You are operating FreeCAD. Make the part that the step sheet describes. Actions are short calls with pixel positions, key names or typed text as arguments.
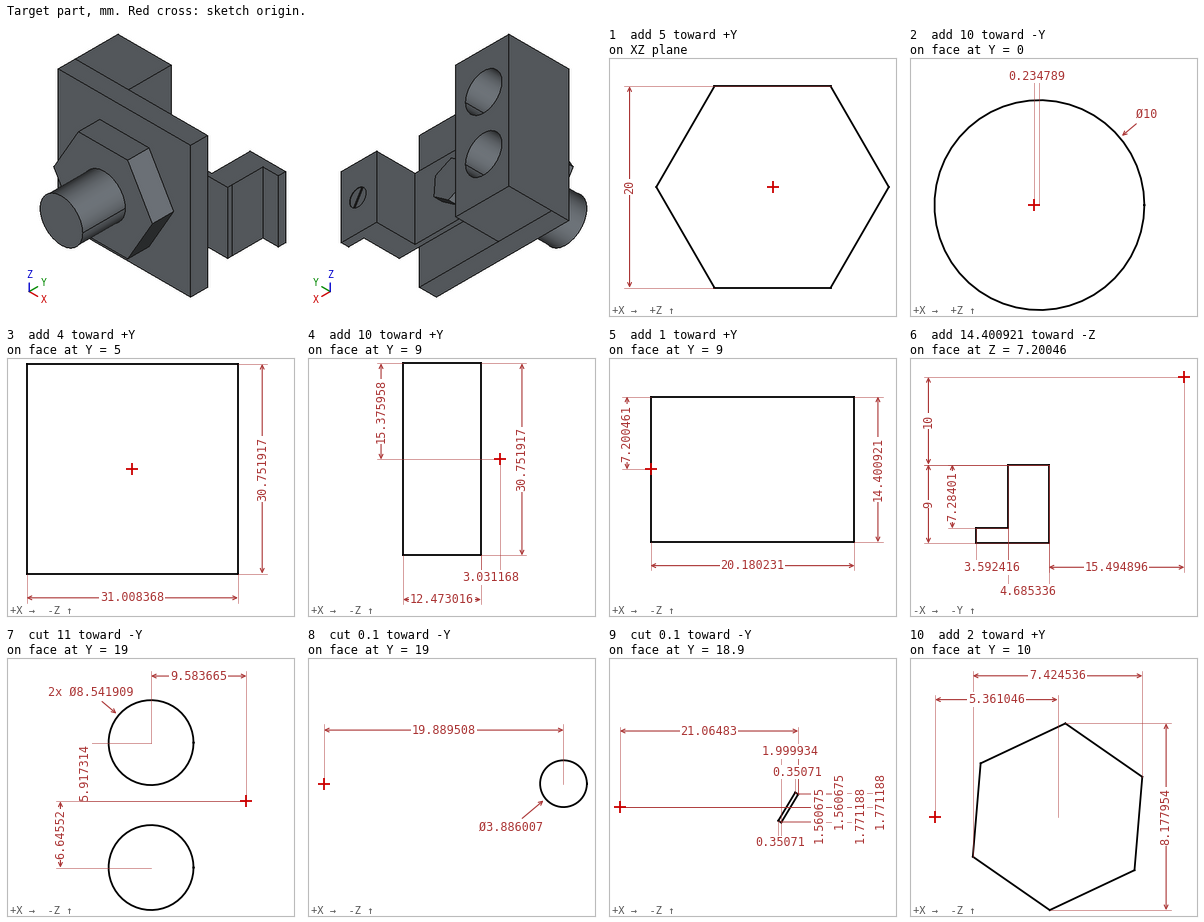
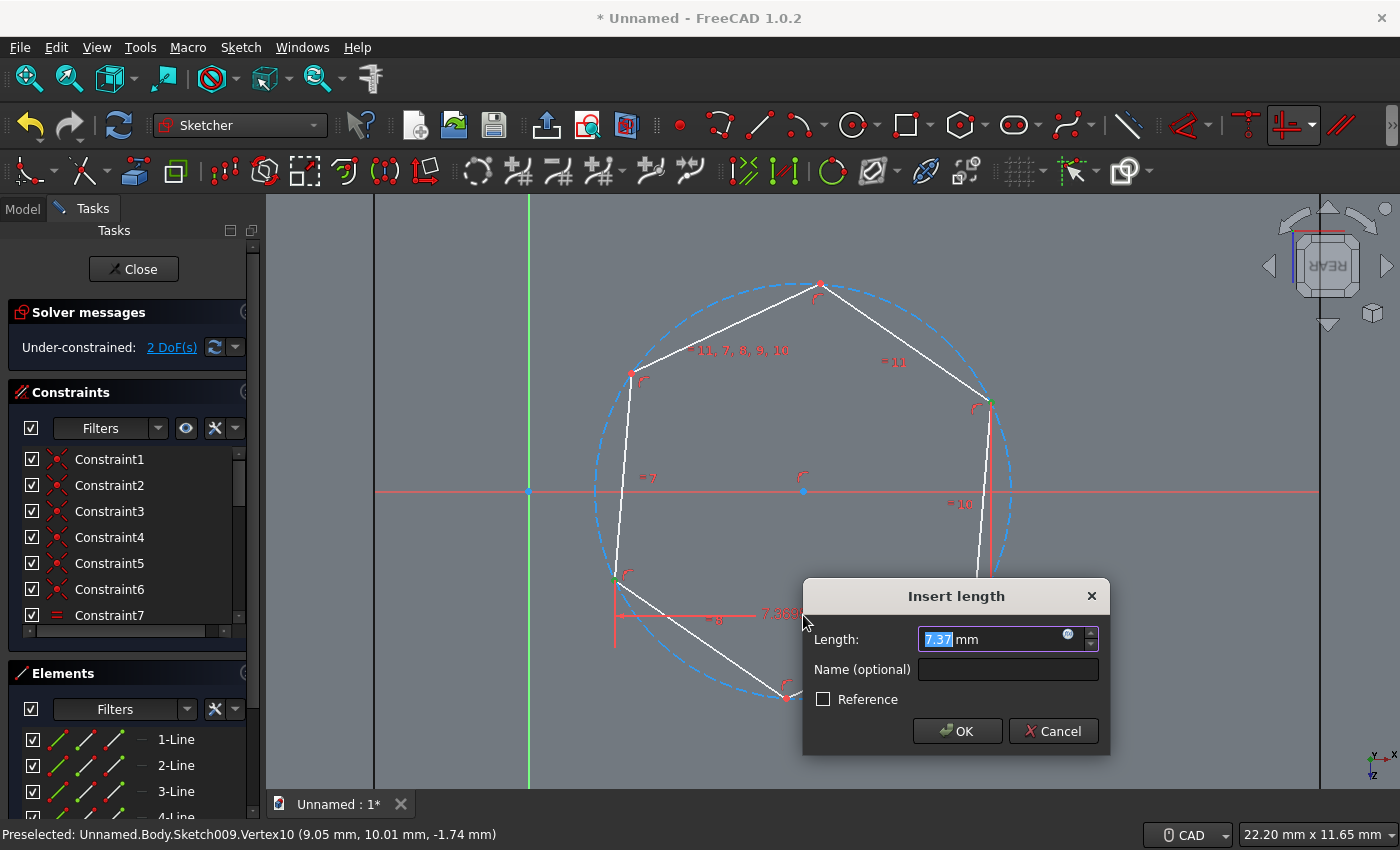
text(7.424536)
key(Return)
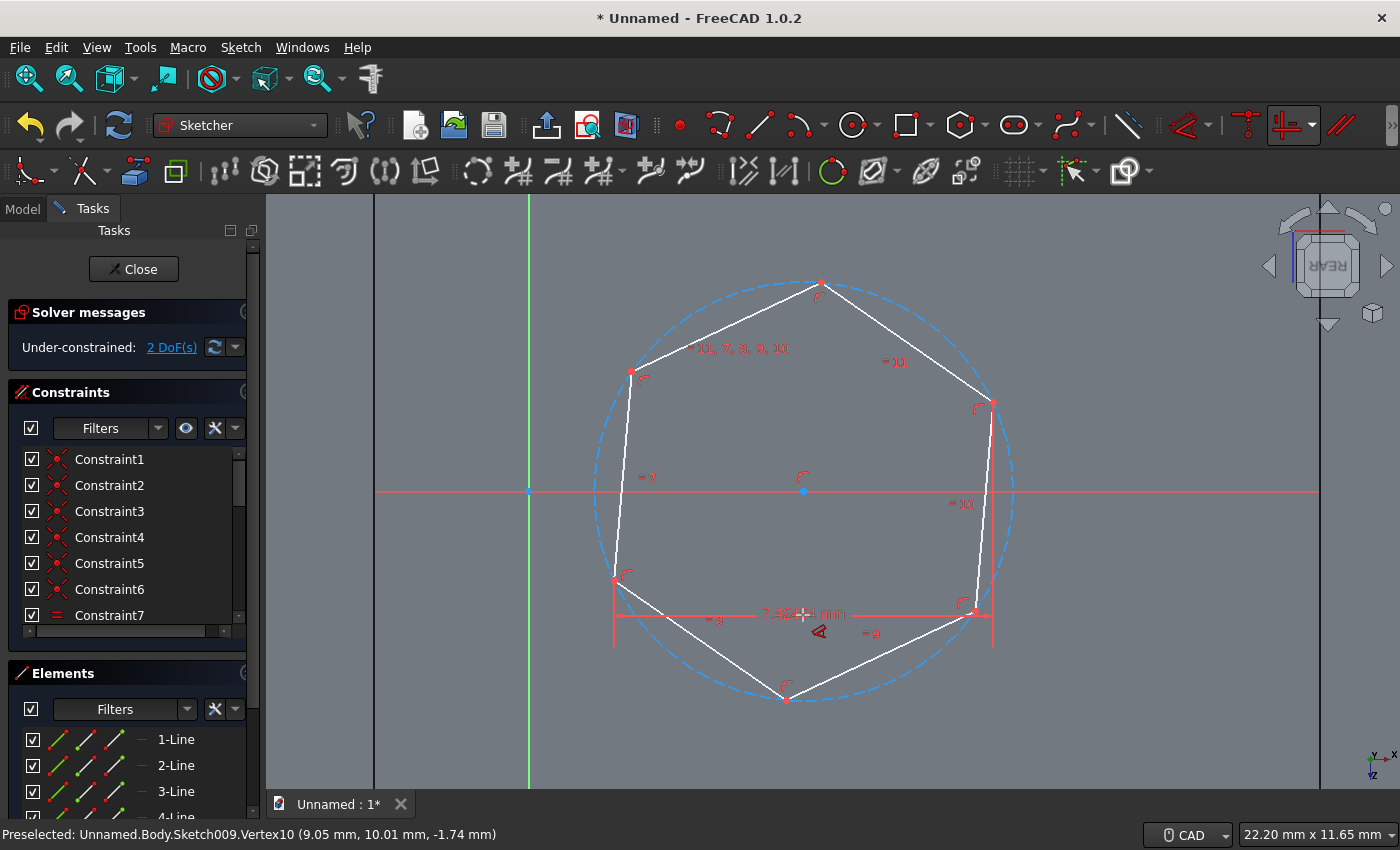
click(786, 700)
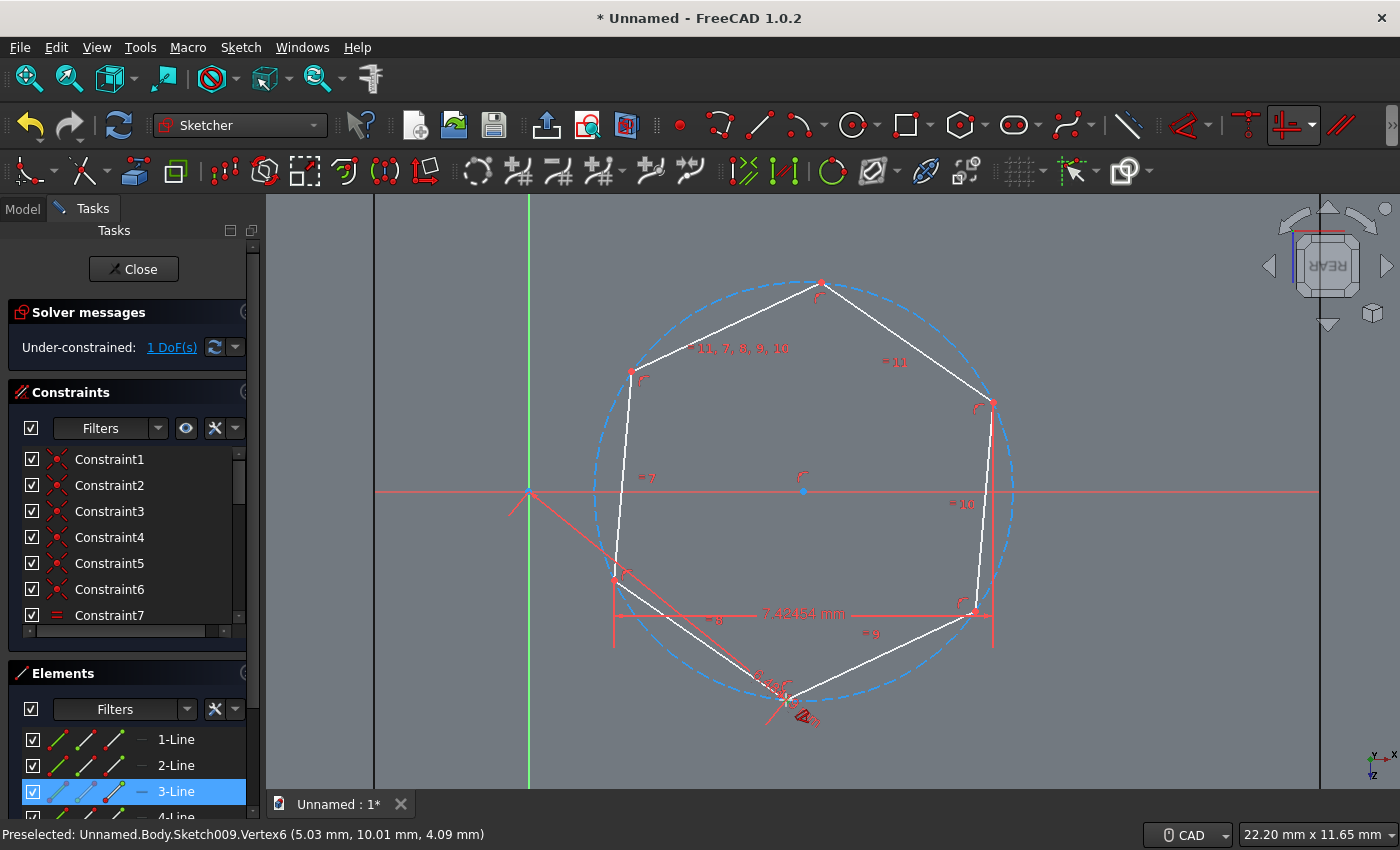
click(821, 283)
click(855, 395)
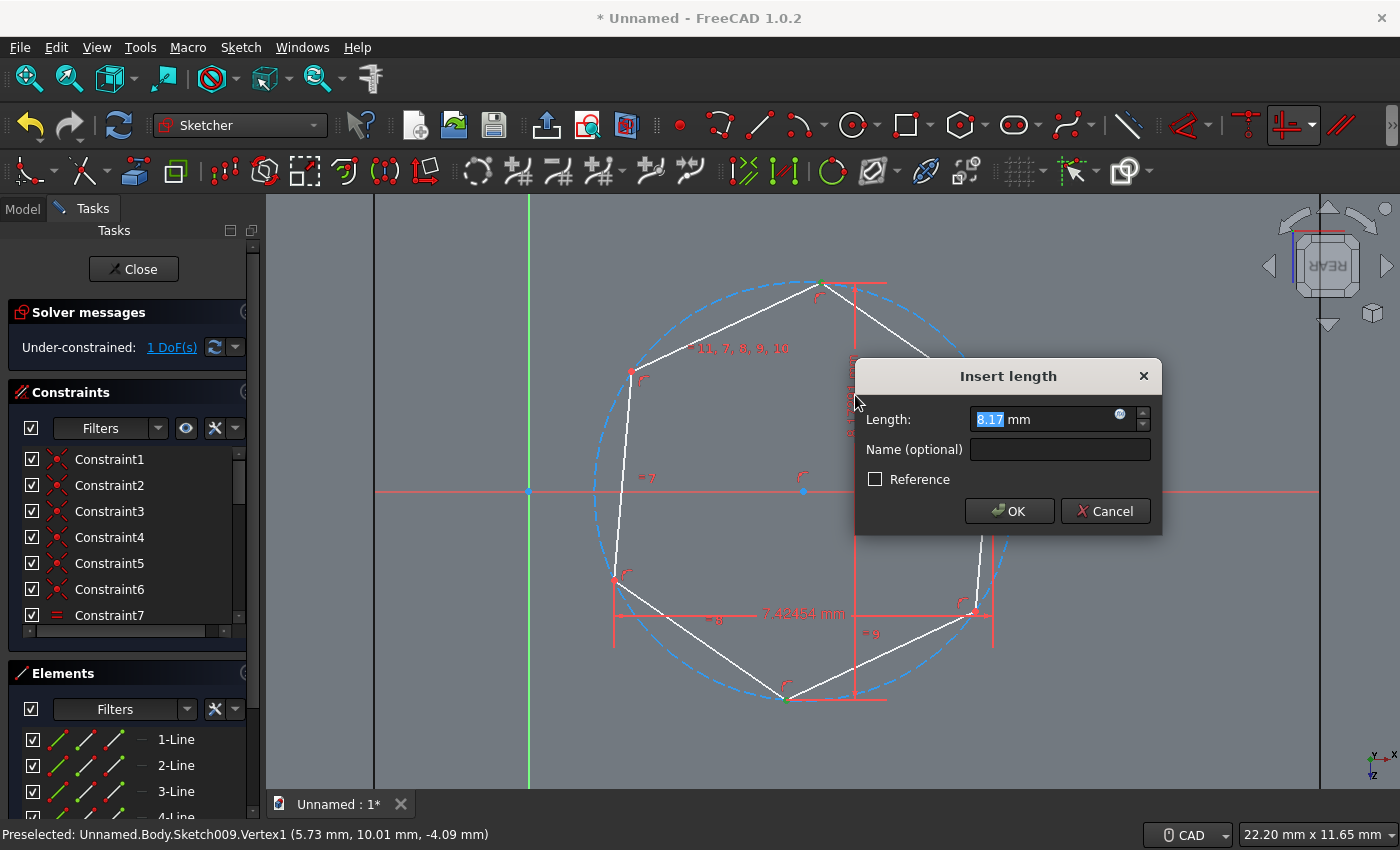
text(8.177954)
key(Return)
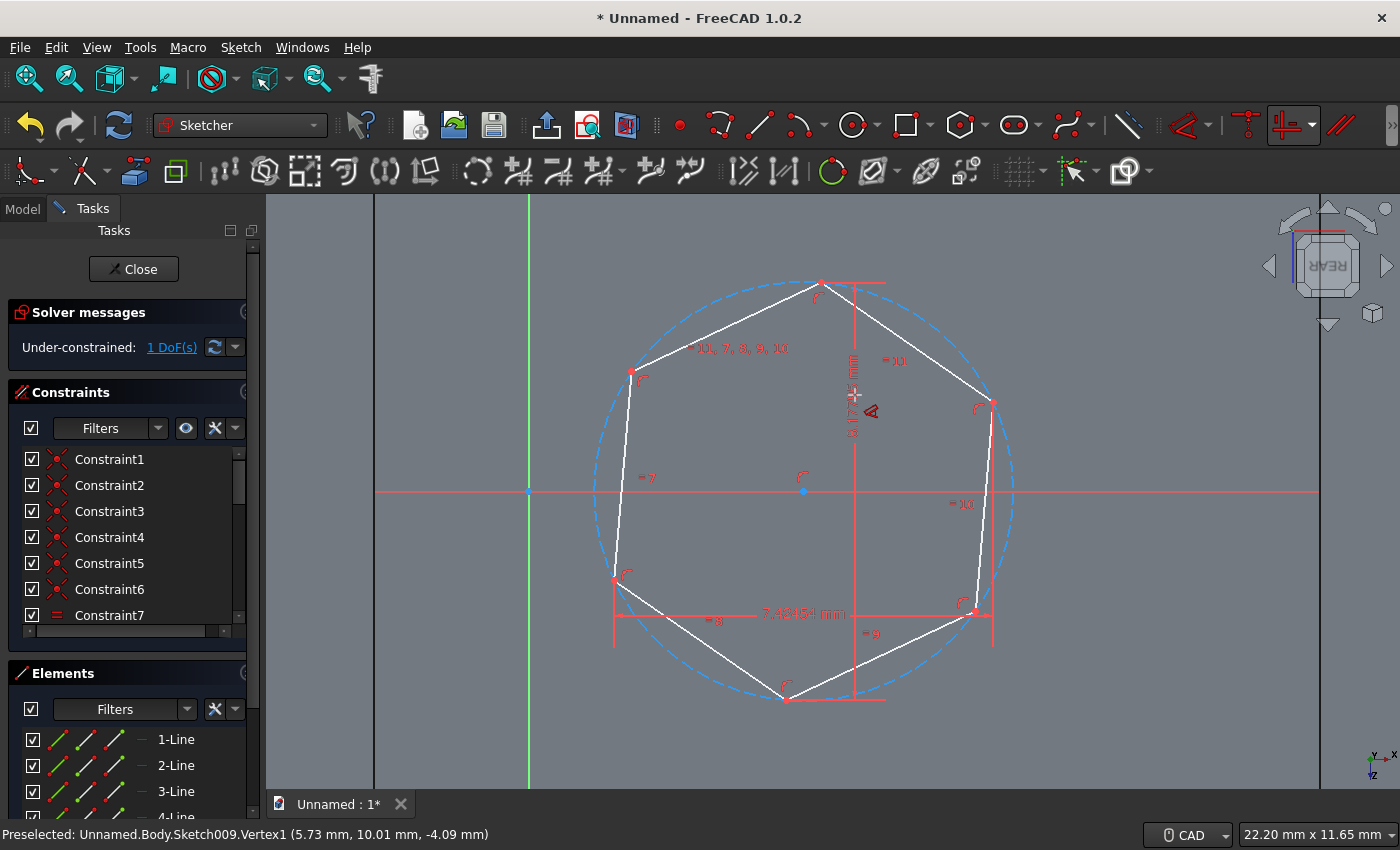
click(804, 491)
click(666, 525)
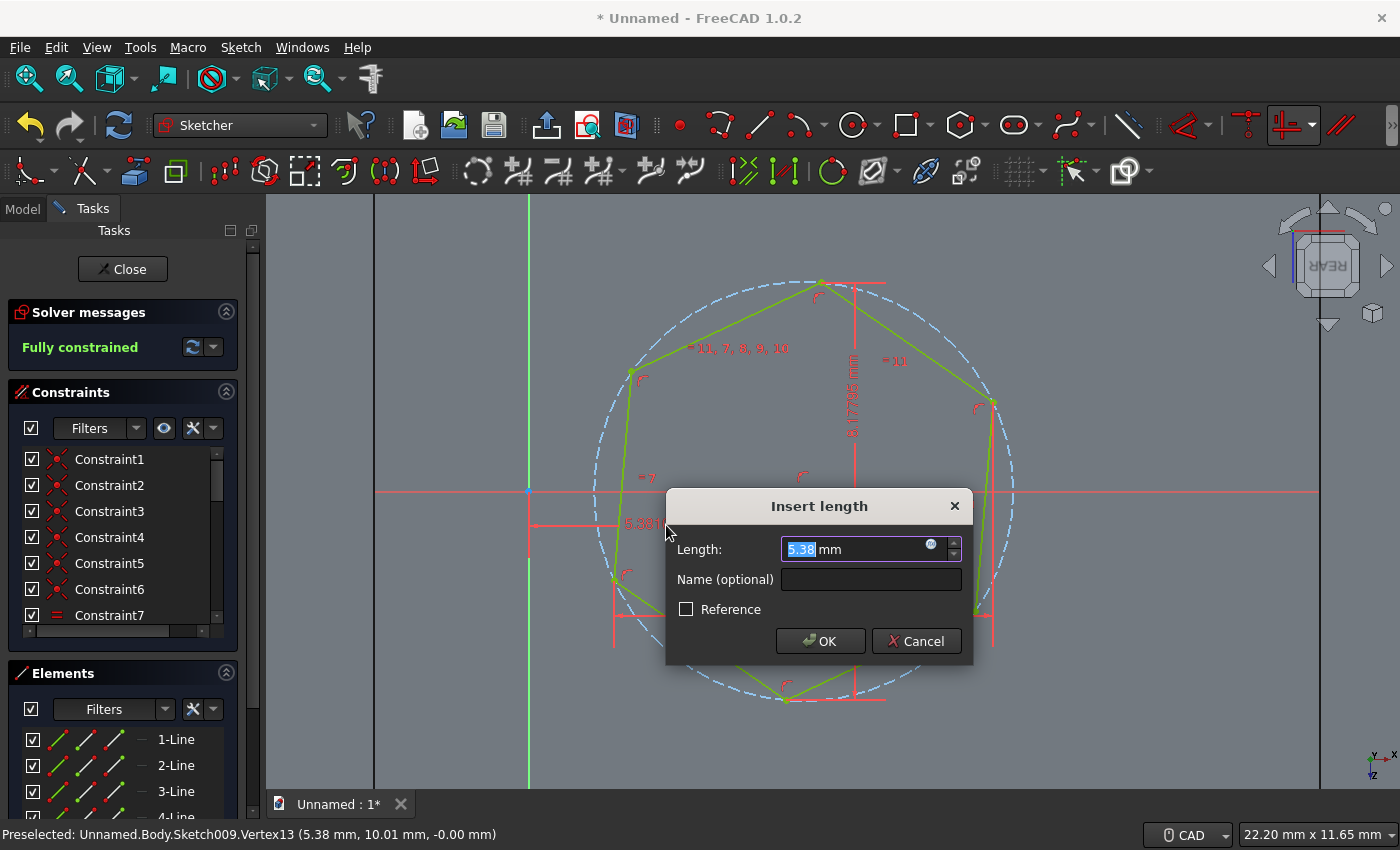
text(5.361046)
key(Return)
key(Escape)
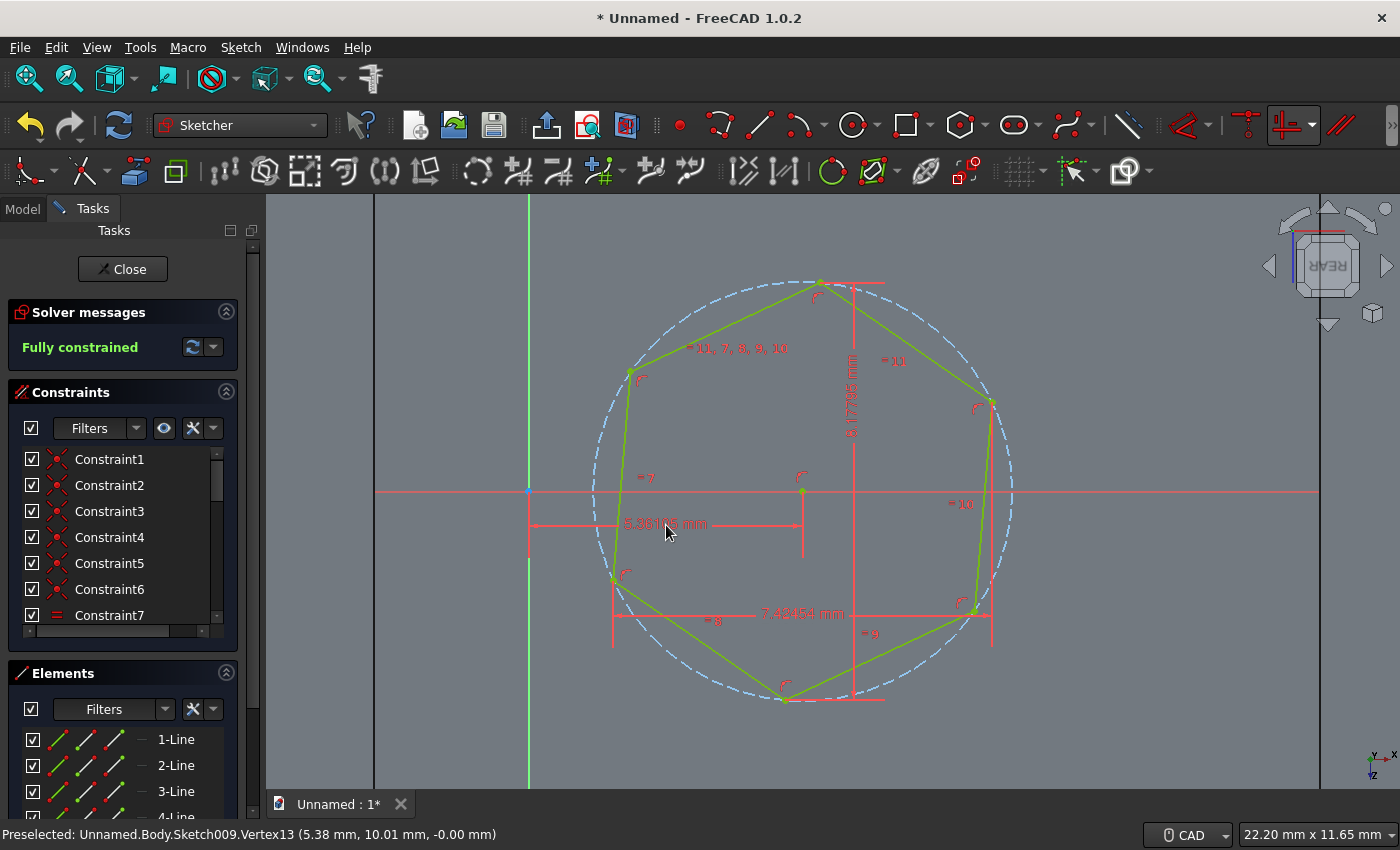
click(123, 269)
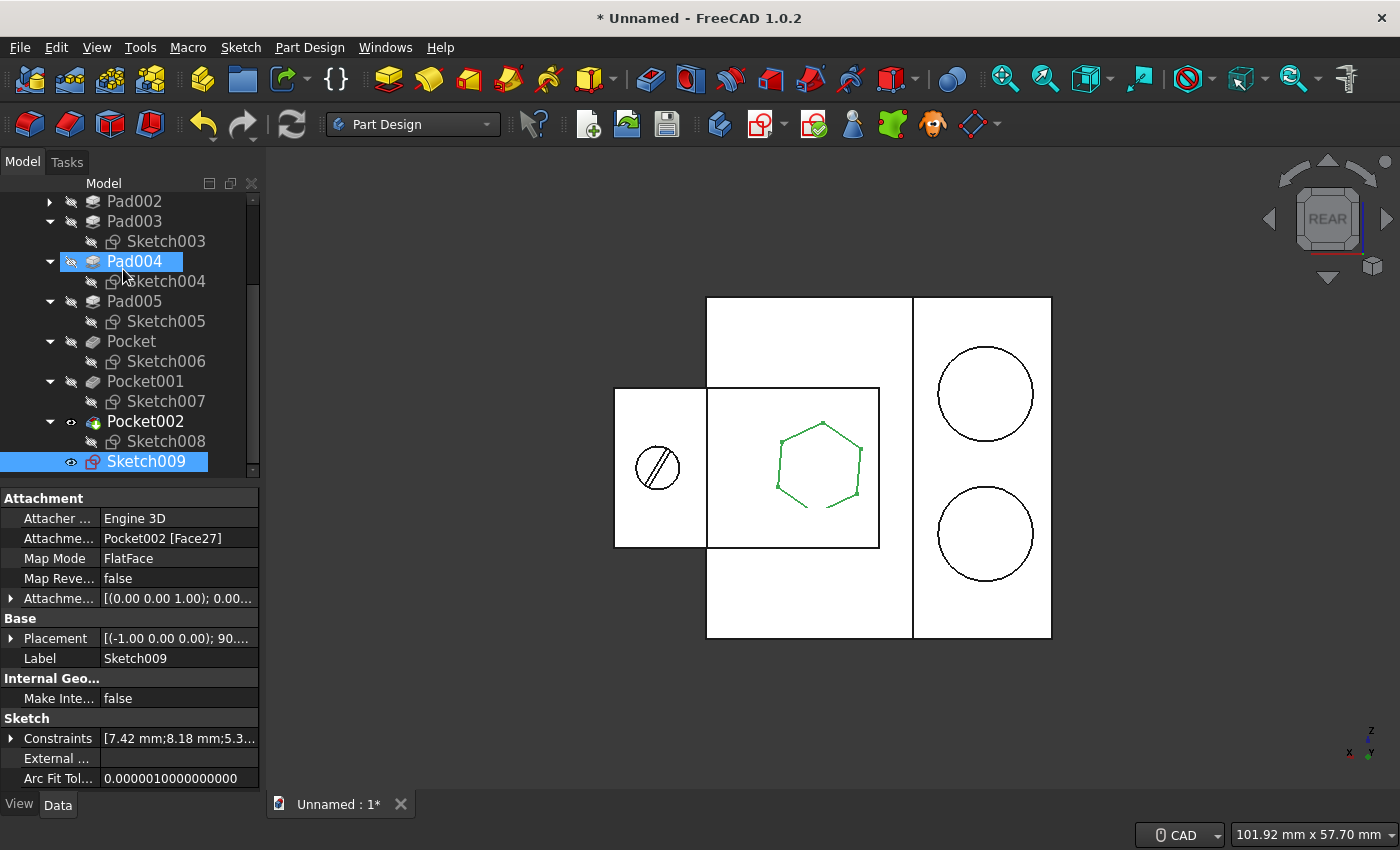
click(390, 80)